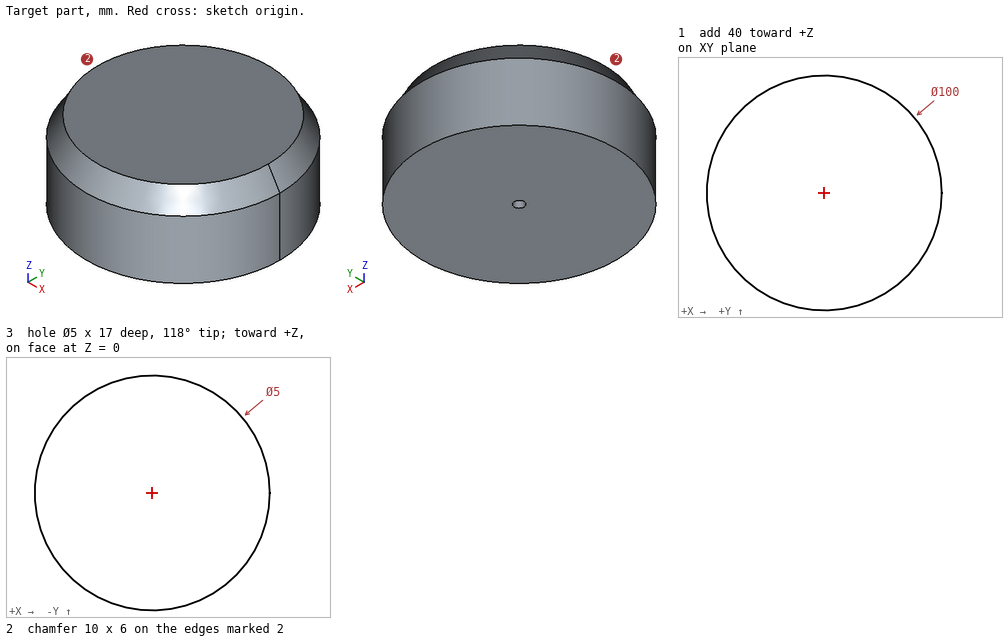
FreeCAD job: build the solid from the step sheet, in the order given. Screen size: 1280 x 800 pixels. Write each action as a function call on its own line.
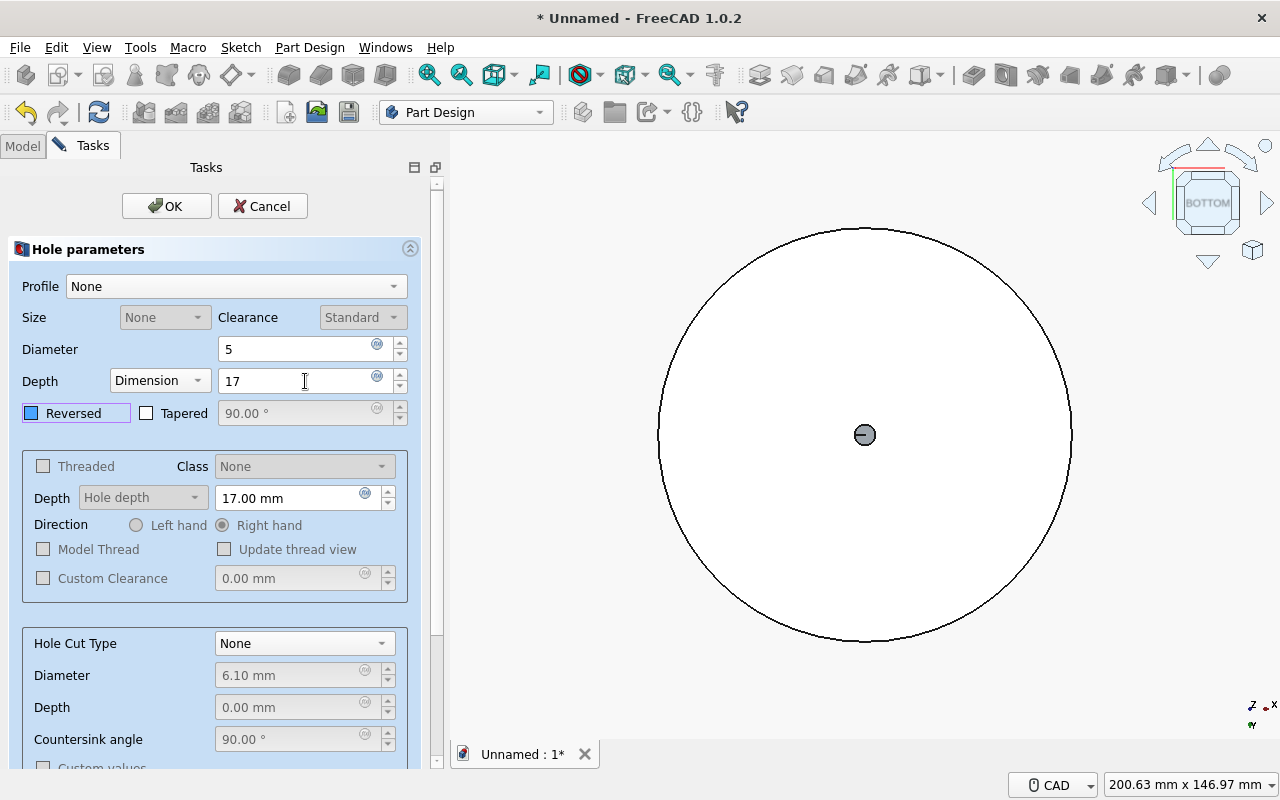
click(167, 206)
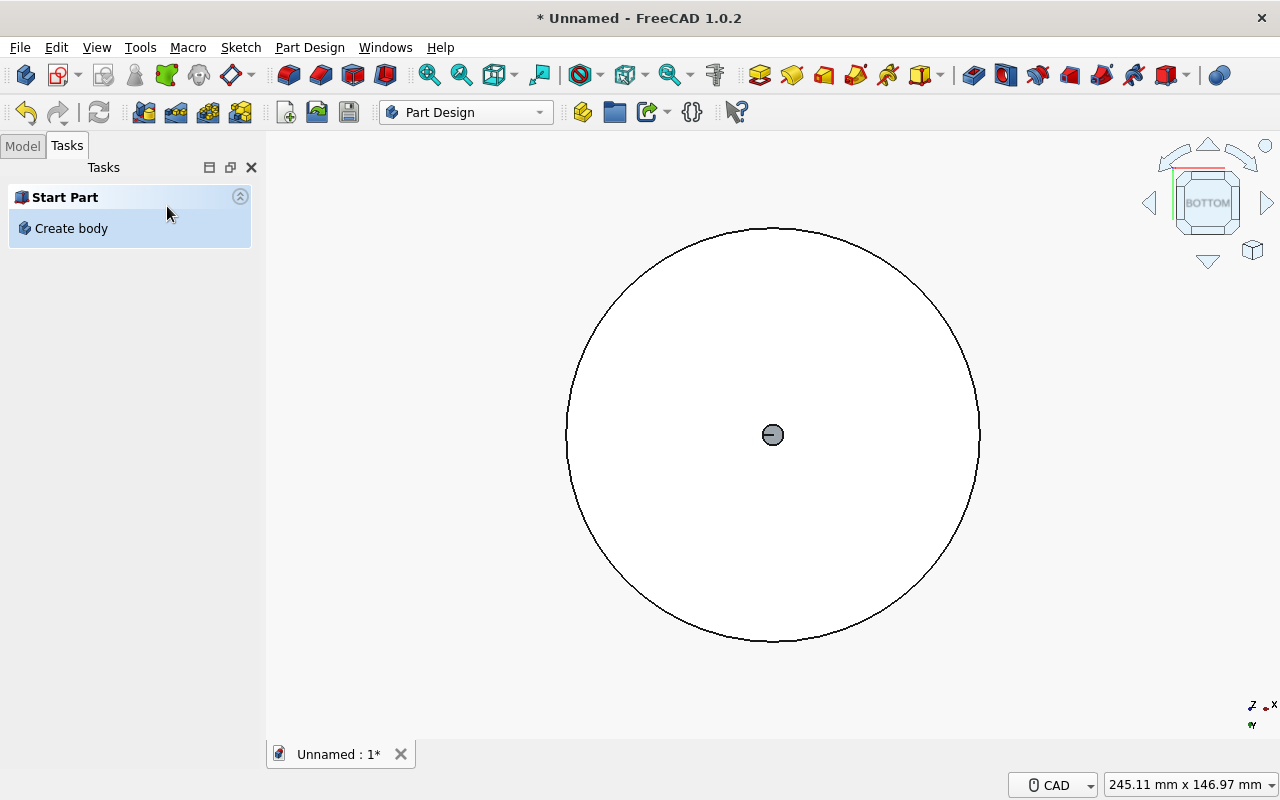
key(0)